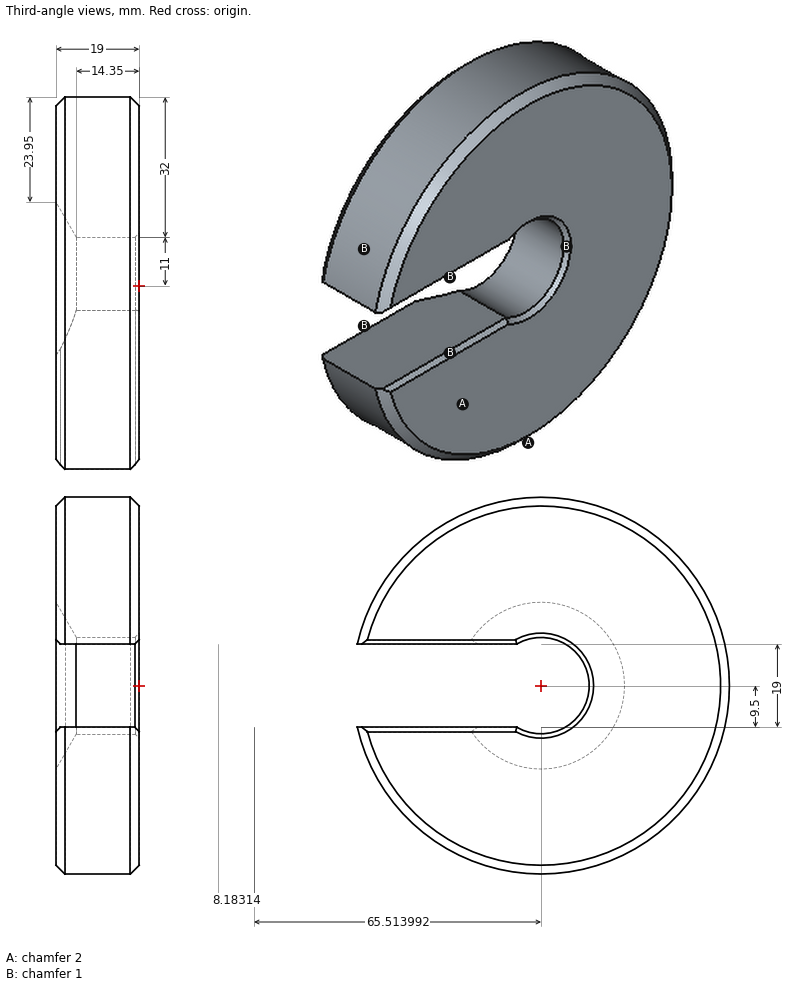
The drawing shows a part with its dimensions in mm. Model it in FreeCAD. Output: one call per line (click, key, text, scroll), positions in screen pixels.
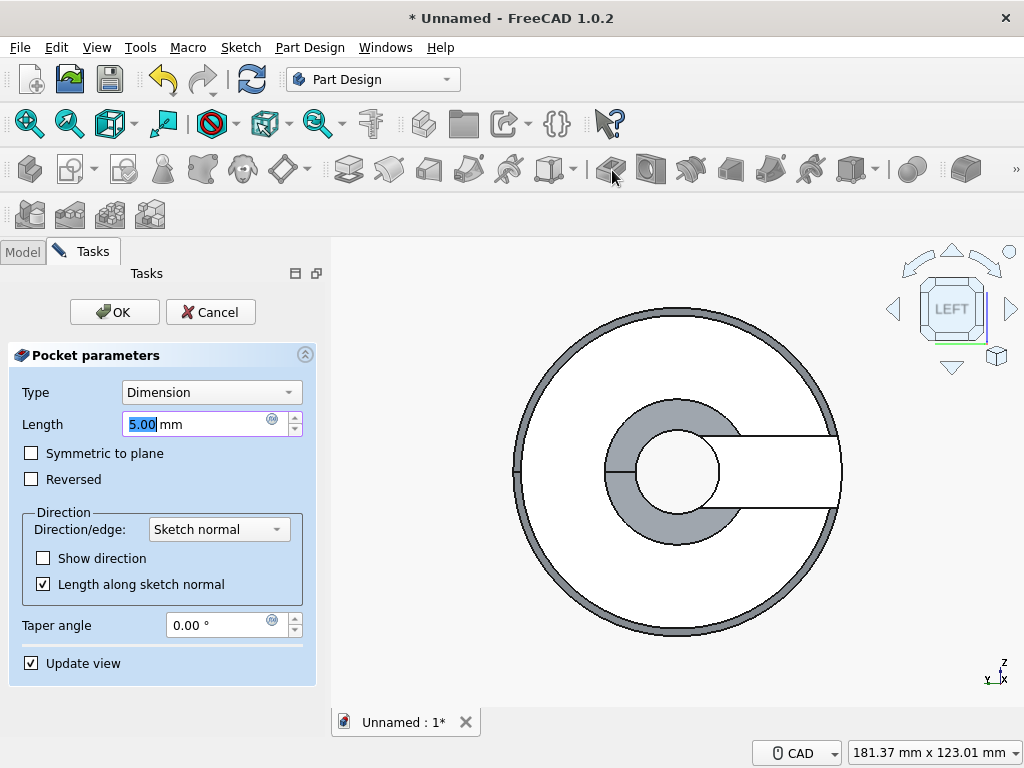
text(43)
key(Tab)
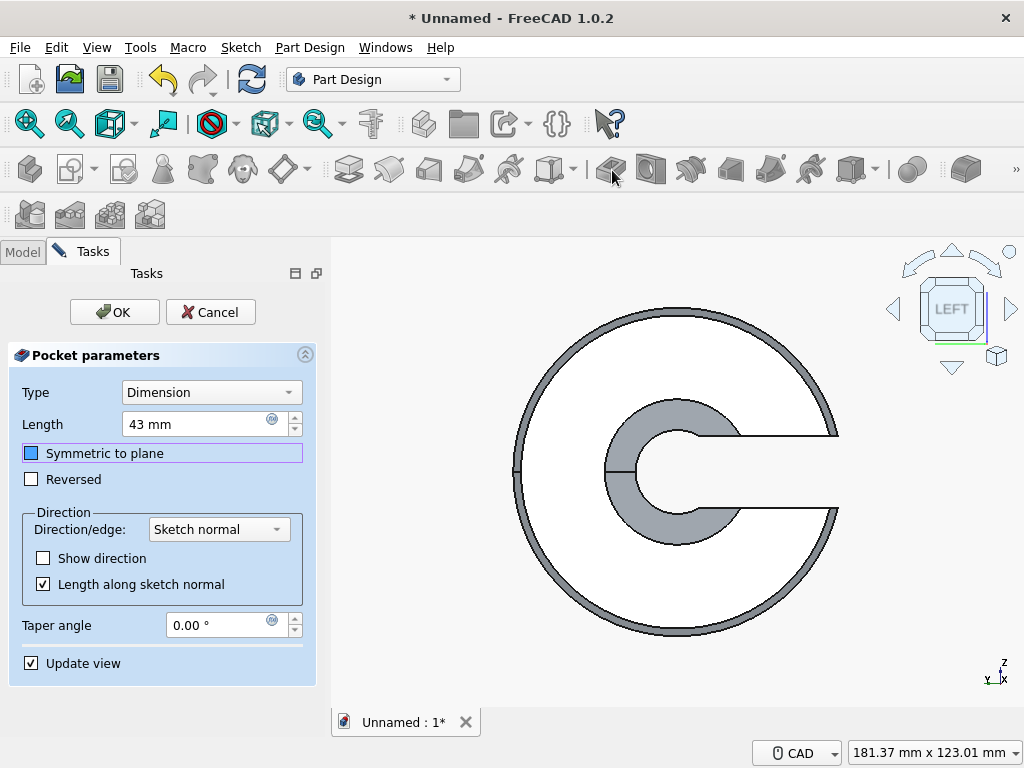
click(115, 312)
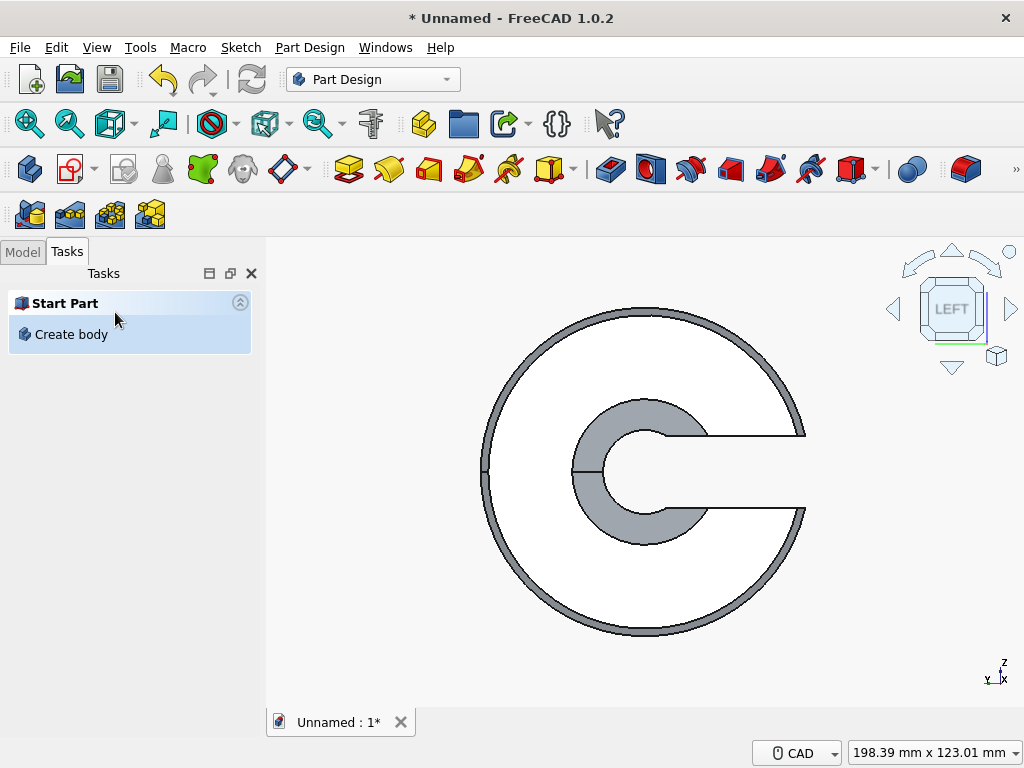
click(753, 507)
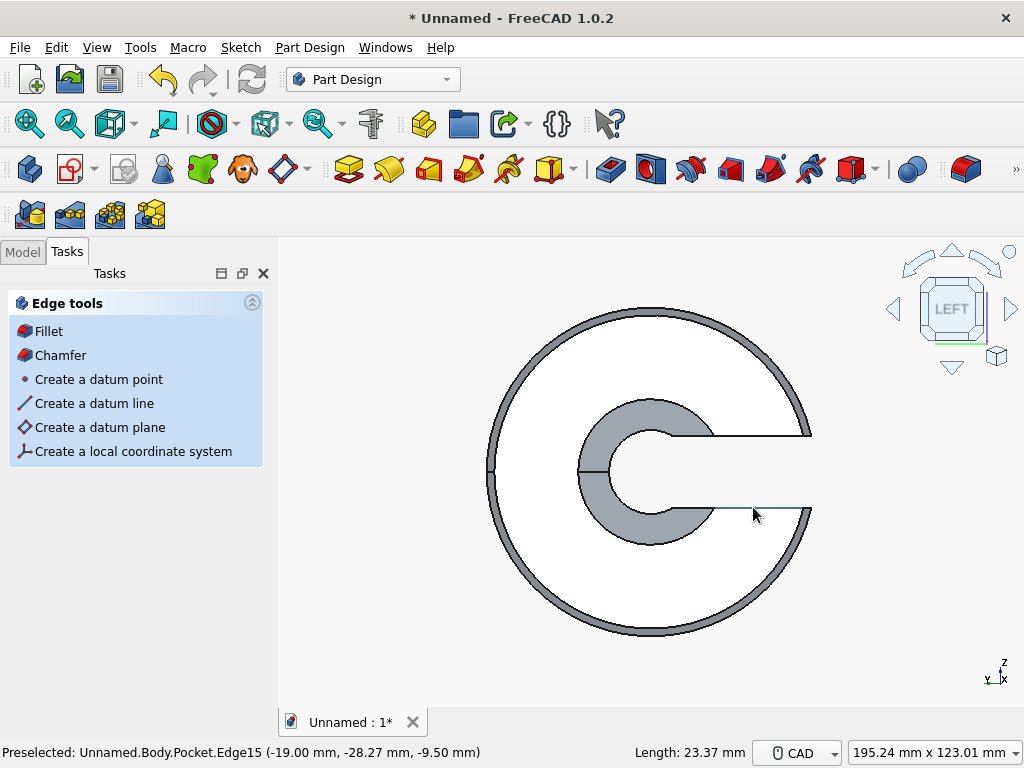
click(759, 435, ctrl)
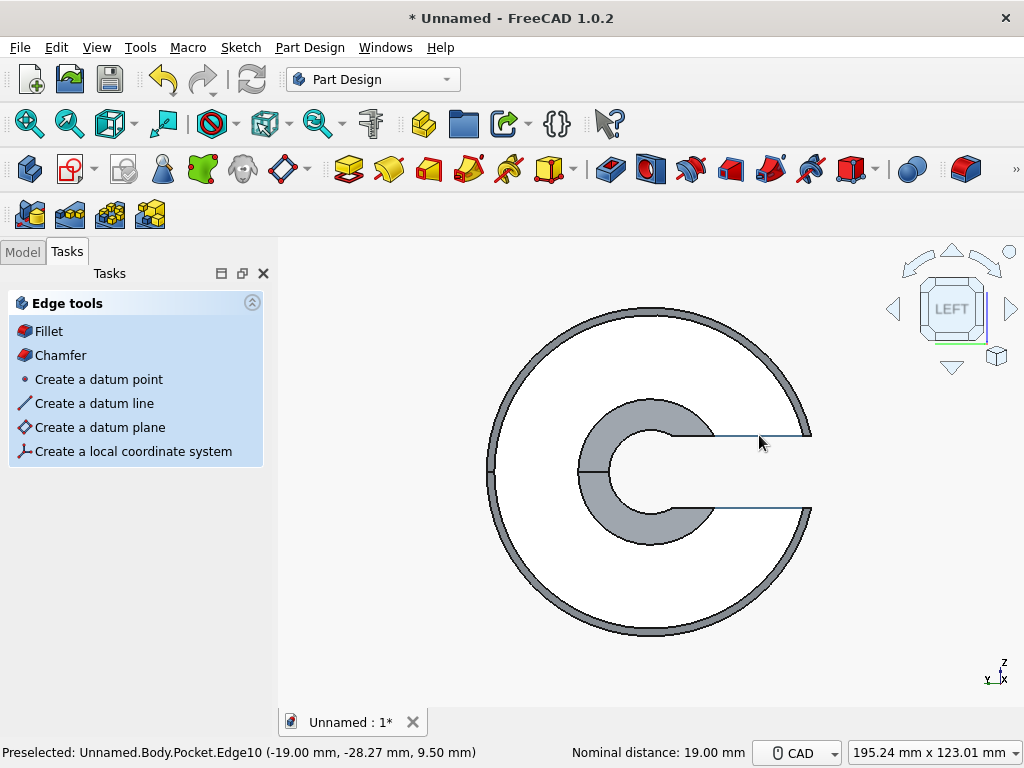
key(0)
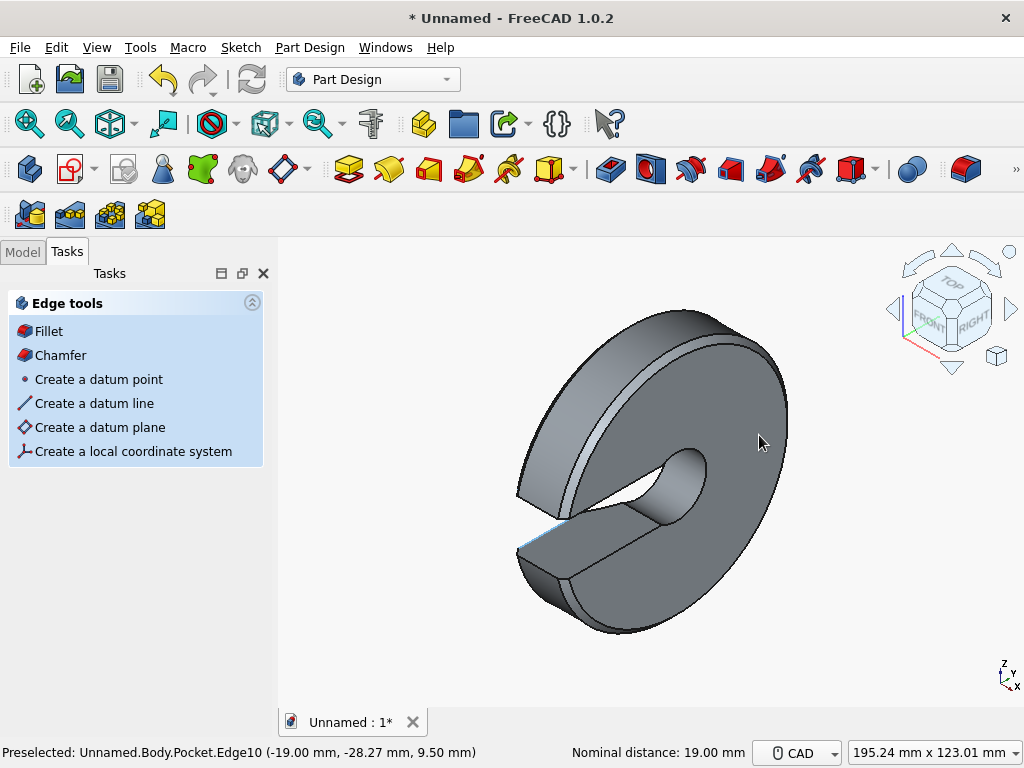
click(615, 551, ctrl)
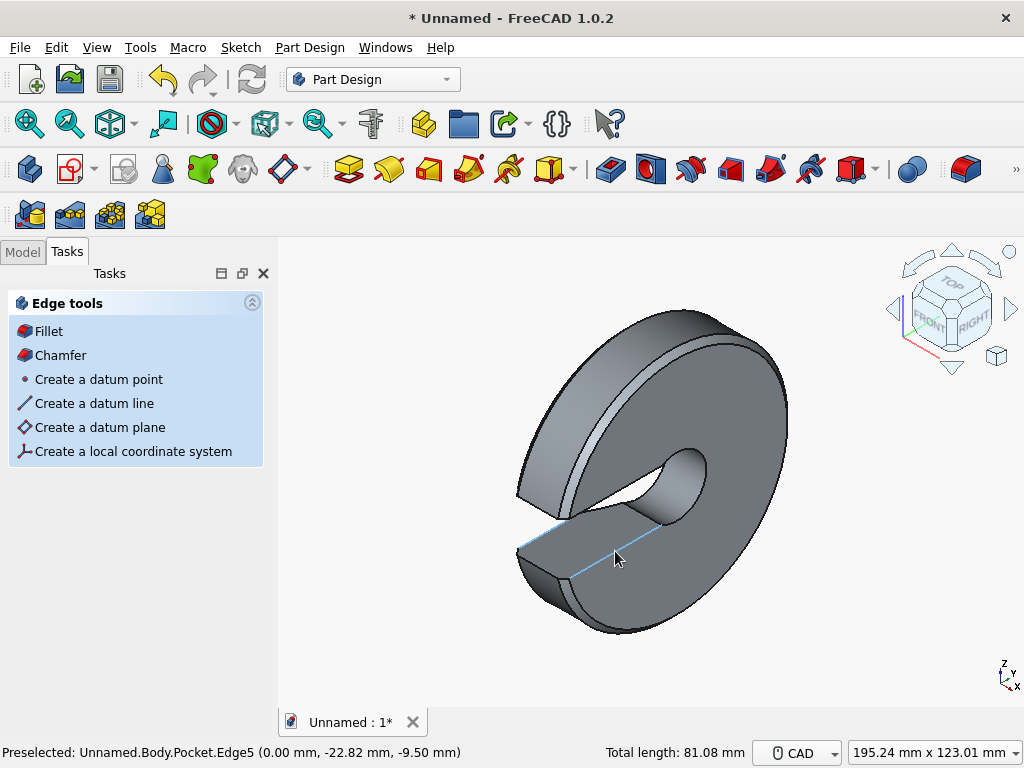
click(701, 452, ctrl)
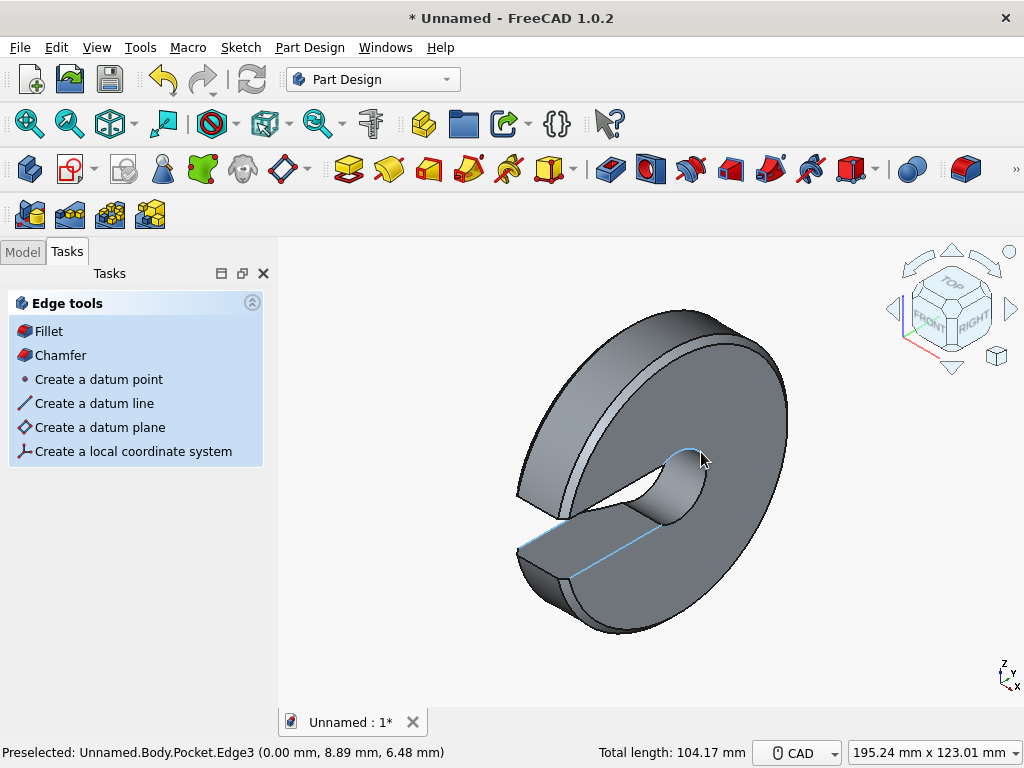
key(2)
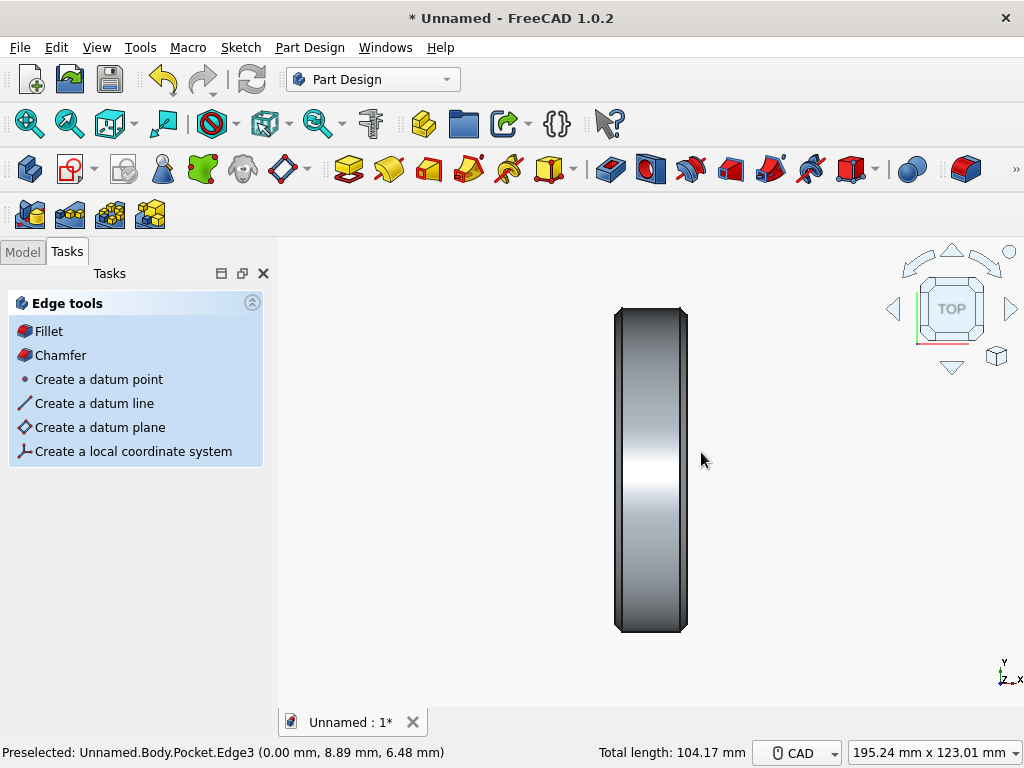
key(1)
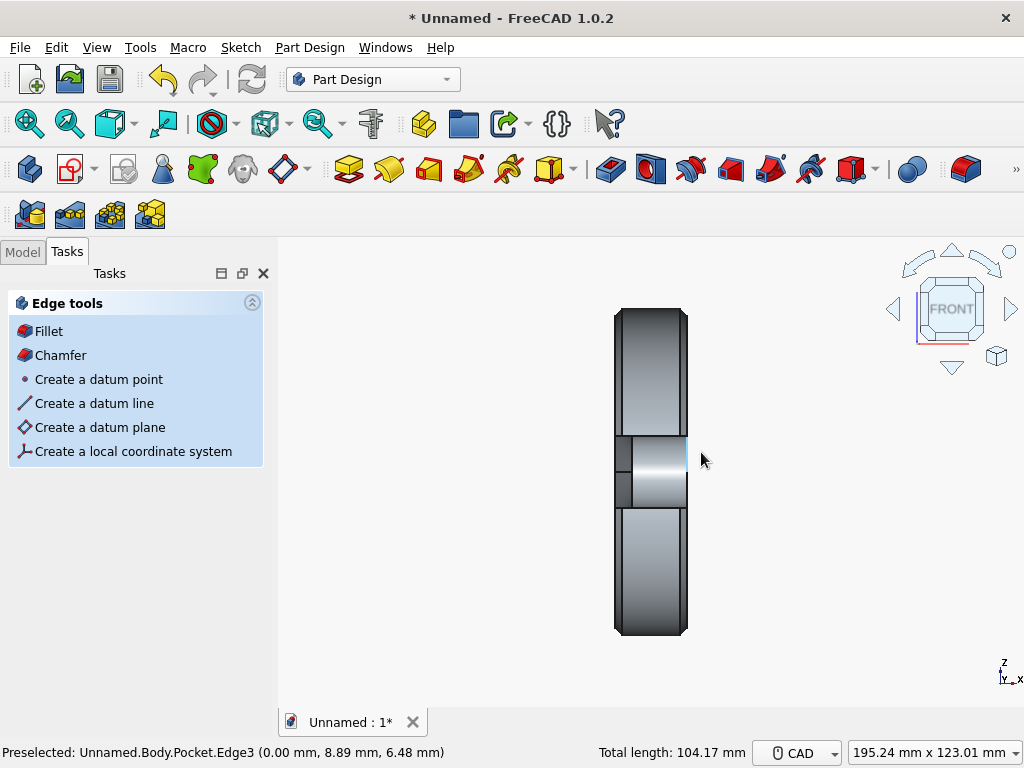
key(3)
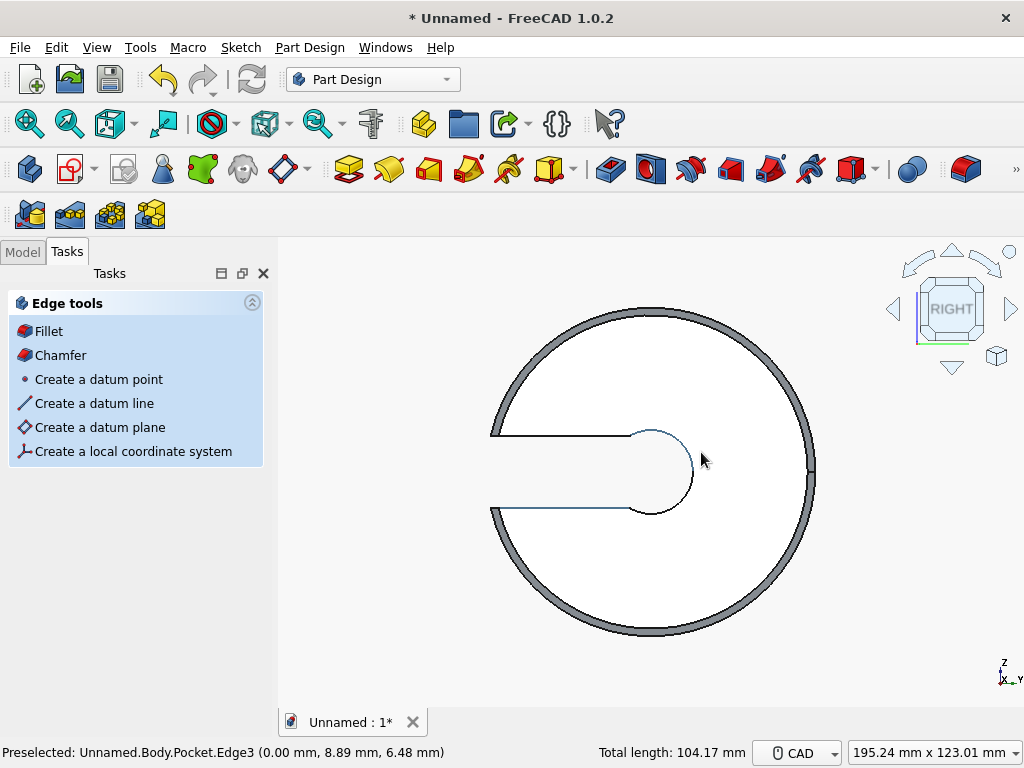
click(564, 435, ctrl)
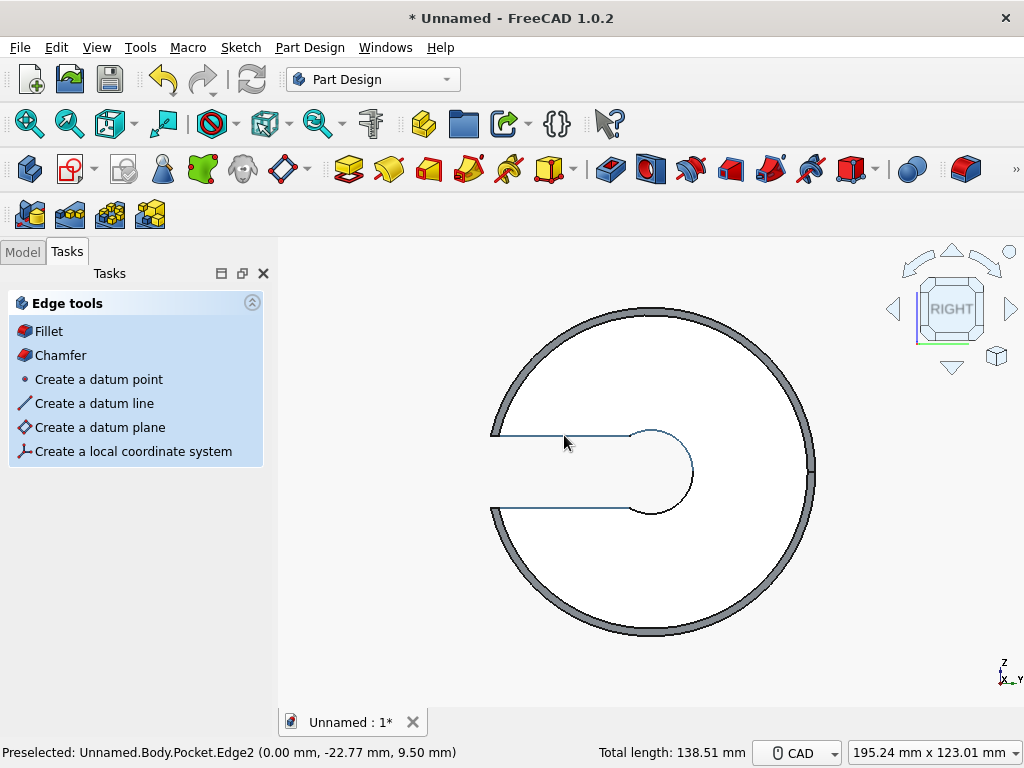
click(136, 355)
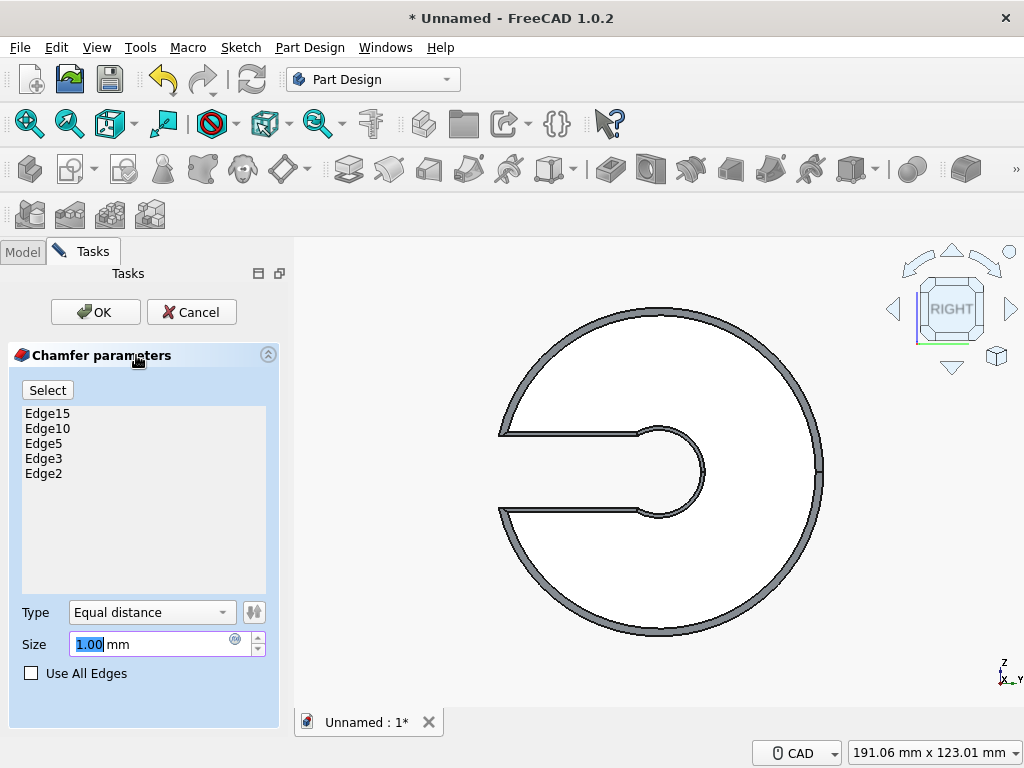
text(1)
key(Tab)